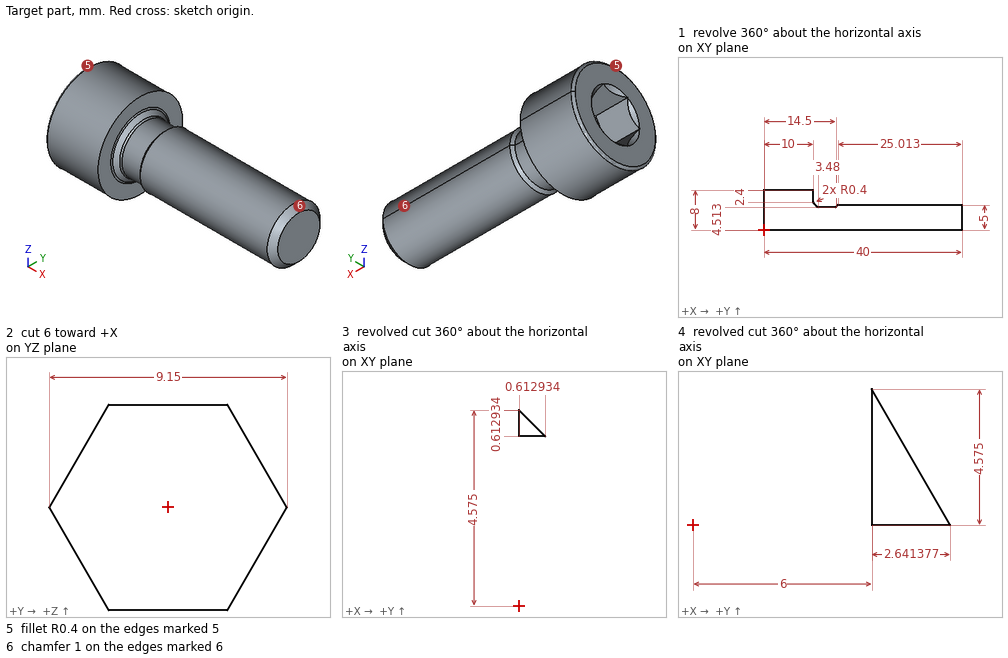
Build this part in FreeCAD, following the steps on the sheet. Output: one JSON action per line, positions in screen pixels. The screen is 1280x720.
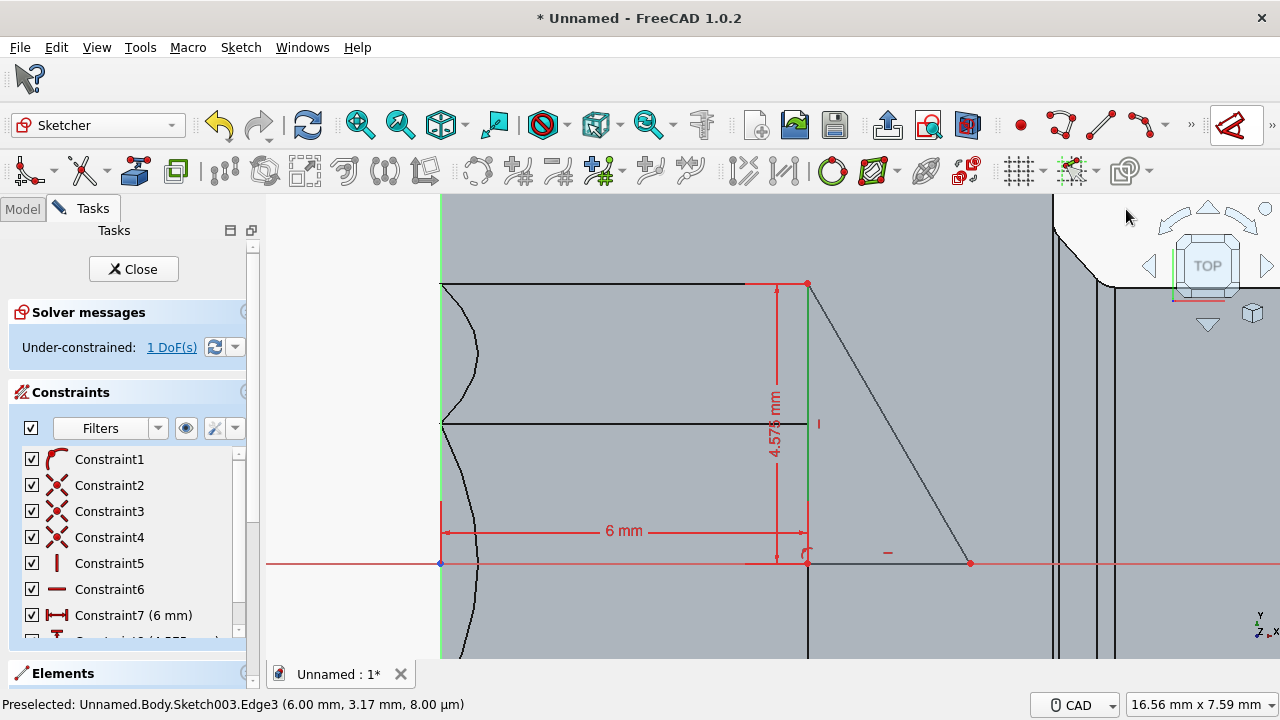
{"action": "left_click", "coordinate": [857, 564]}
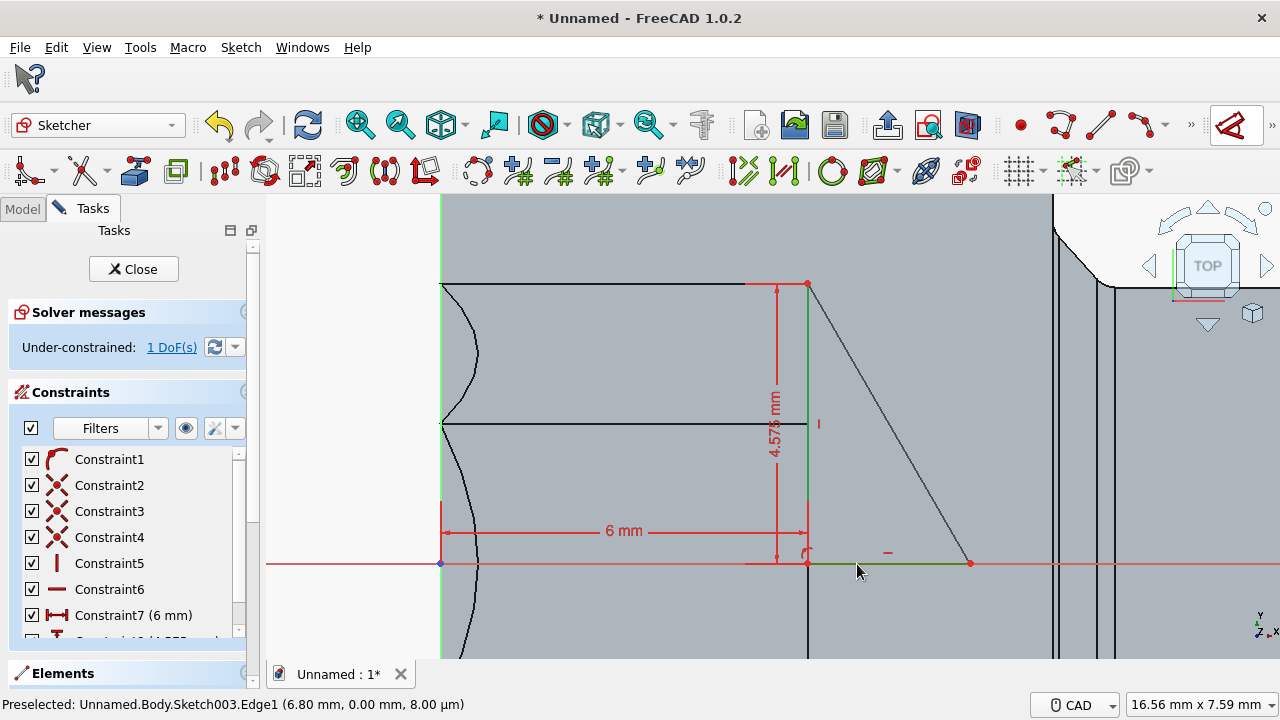
{"action": "left_click", "coordinate": [1258, 126]}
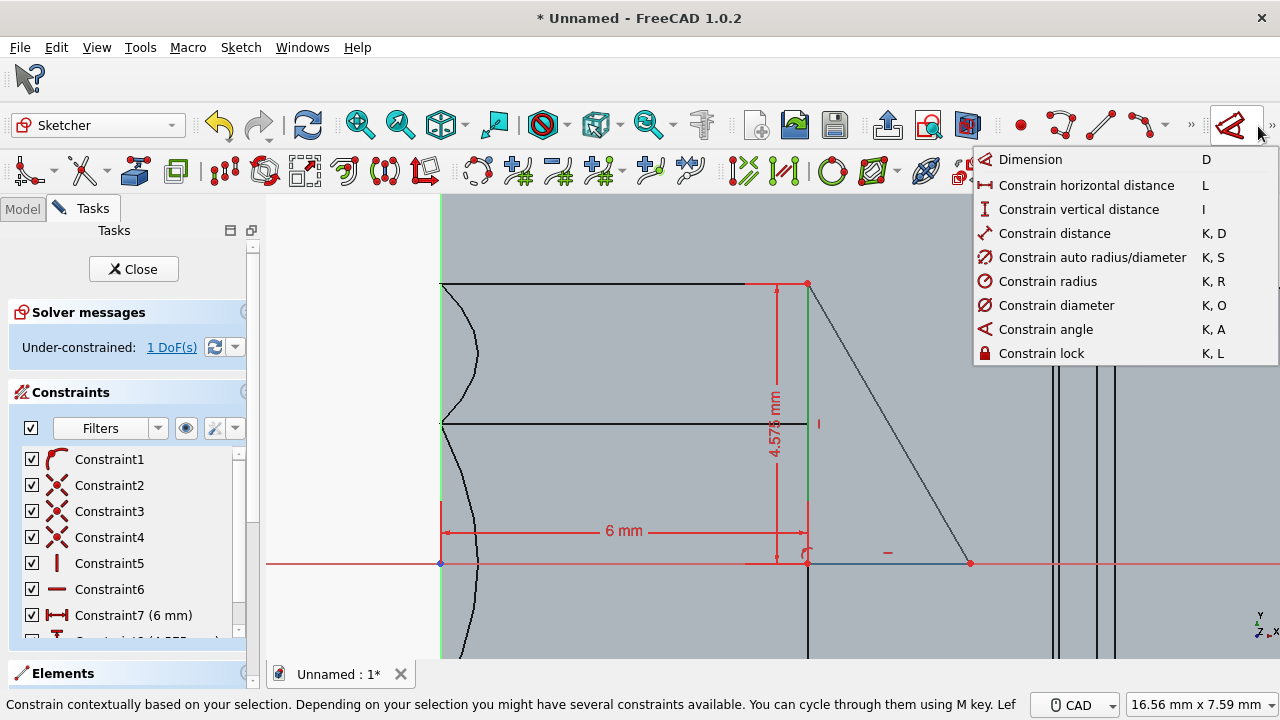
{"action": "left_click", "coordinate": [1126, 185]}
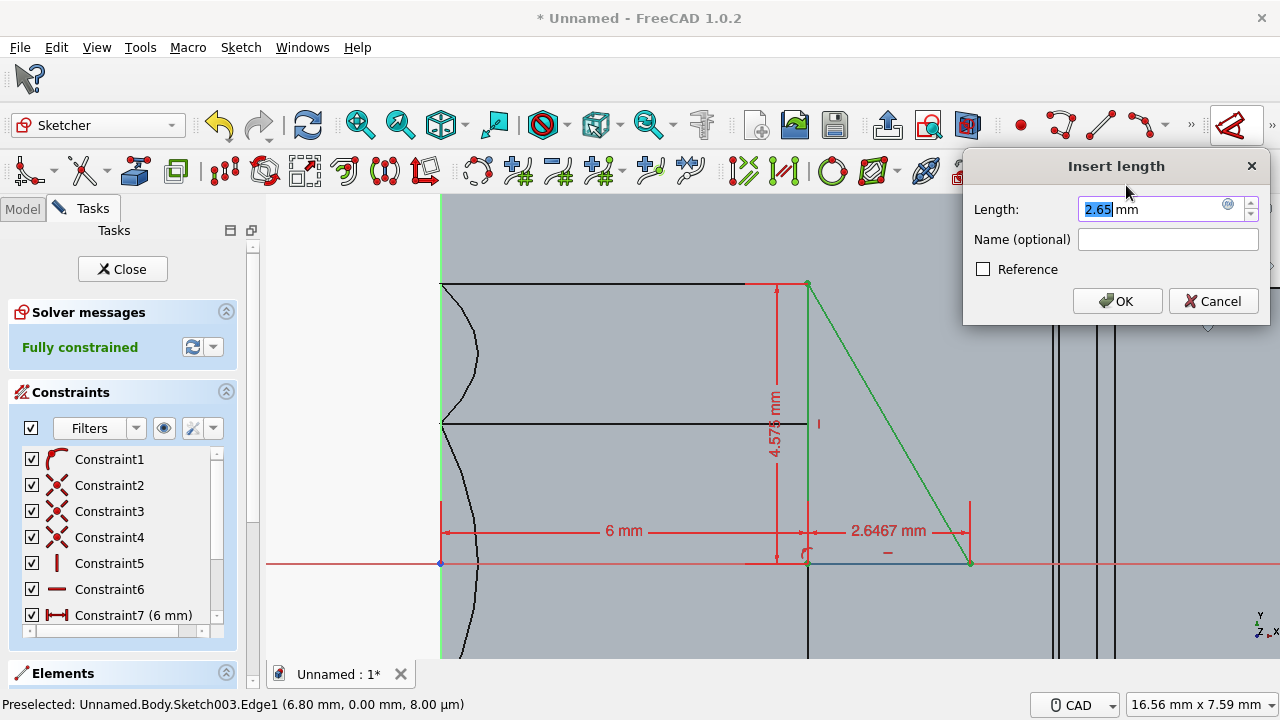
{"action": "type", "text": "2.641377"}
{"action": "key", "text": "Return"}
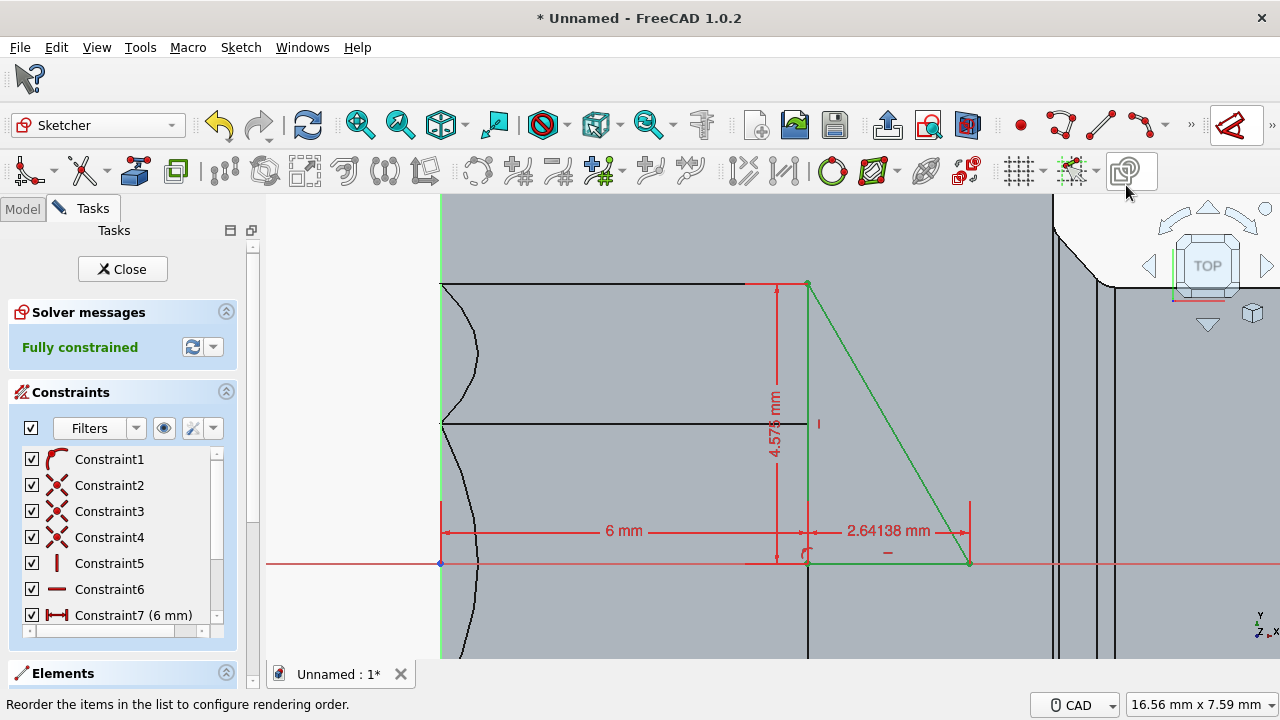
{"action": "left_click", "coordinate": [123, 269]}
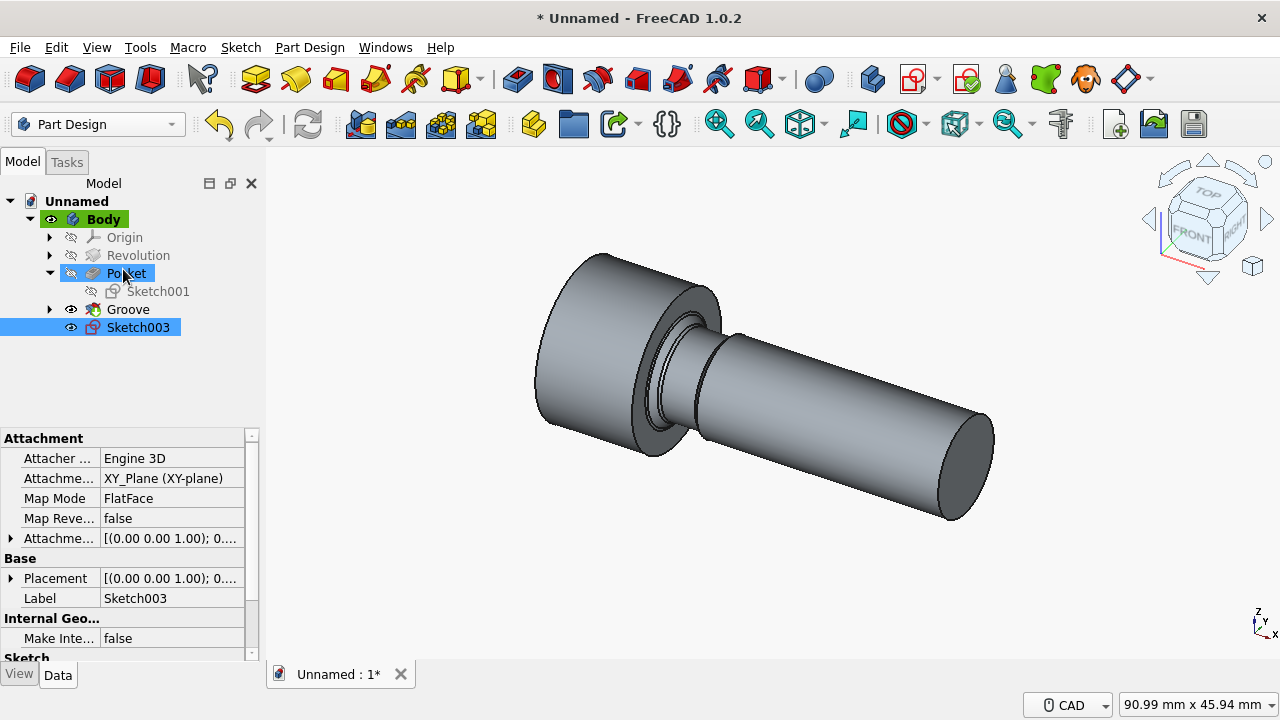
{"action": "left_click", "coordinate": [598, 80]}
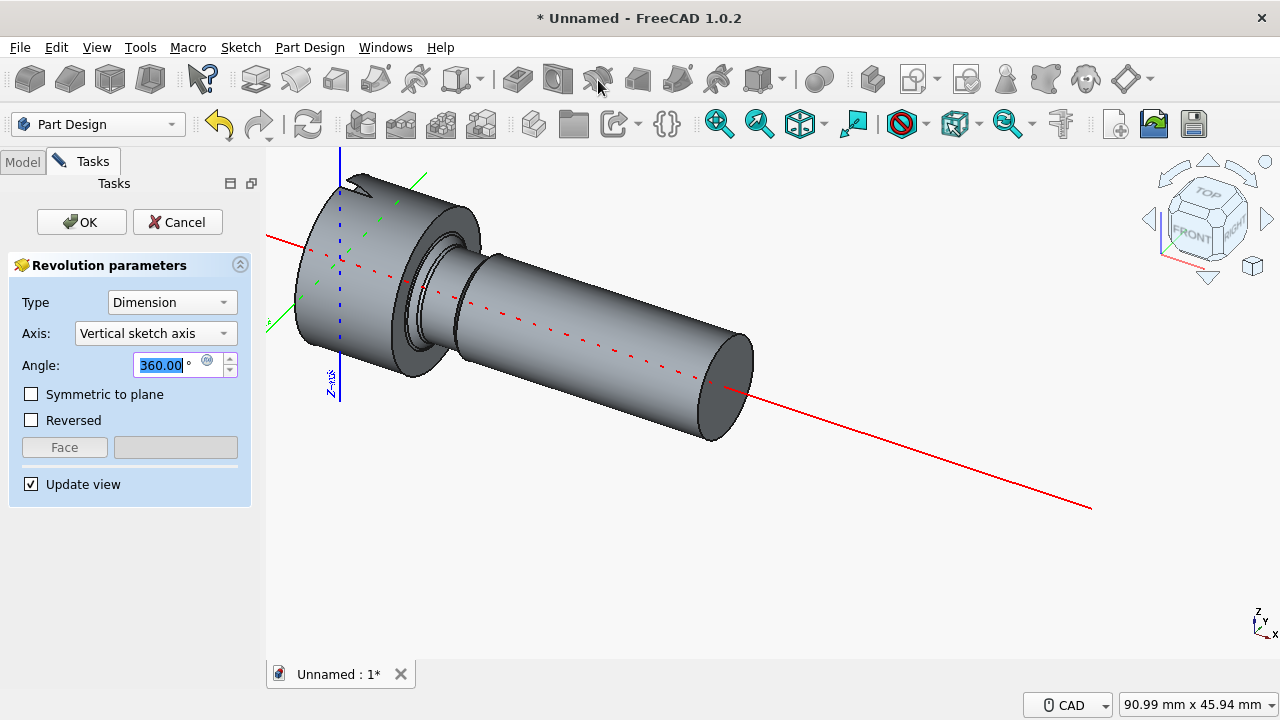
{"action": "left_click", "coordinate": [156, 334]}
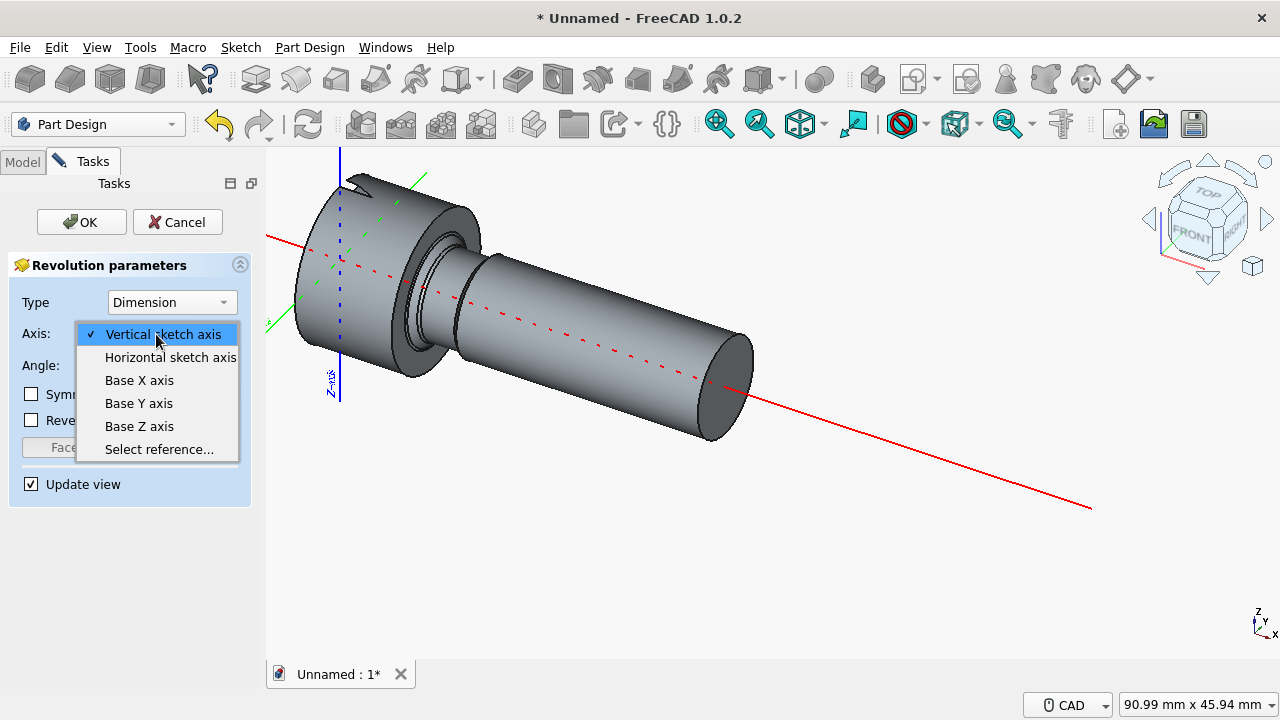
{"action": "left_click", "coordinate": [156, 358]}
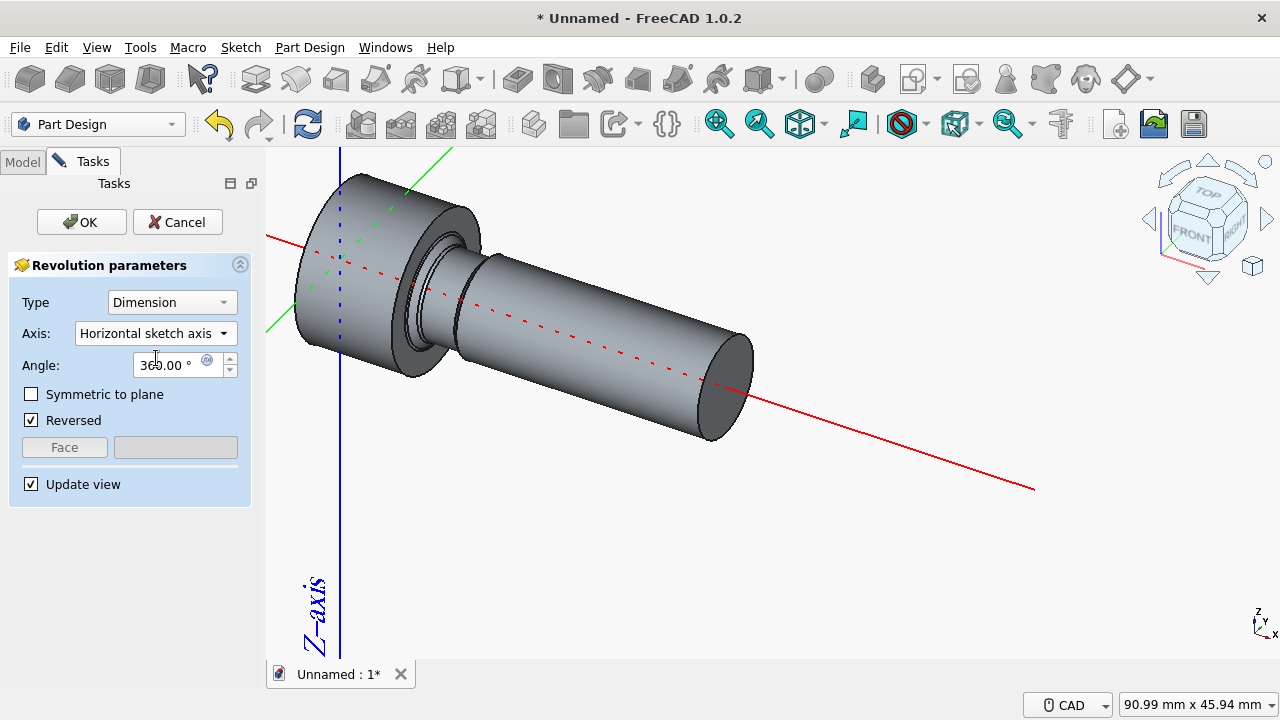
{"action": "left_click", "coordinate": [82, 222]}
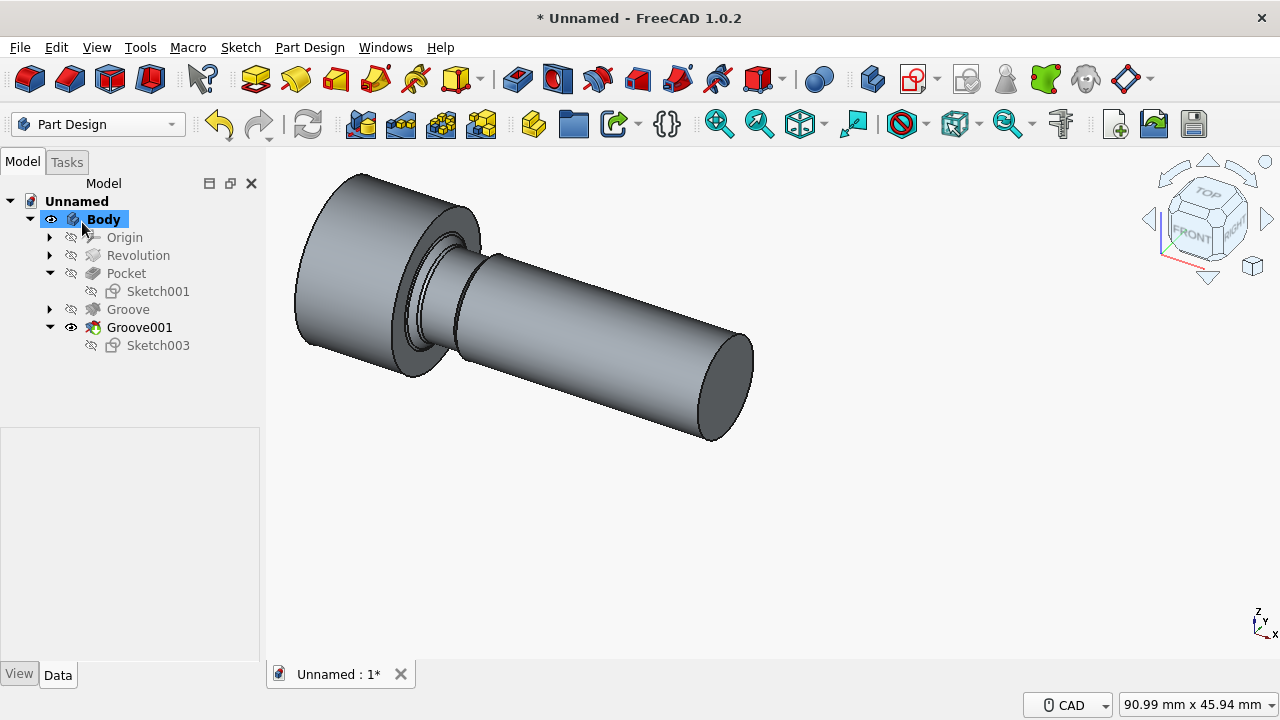
{"action": "left_click", "coordinate": [720, 124]}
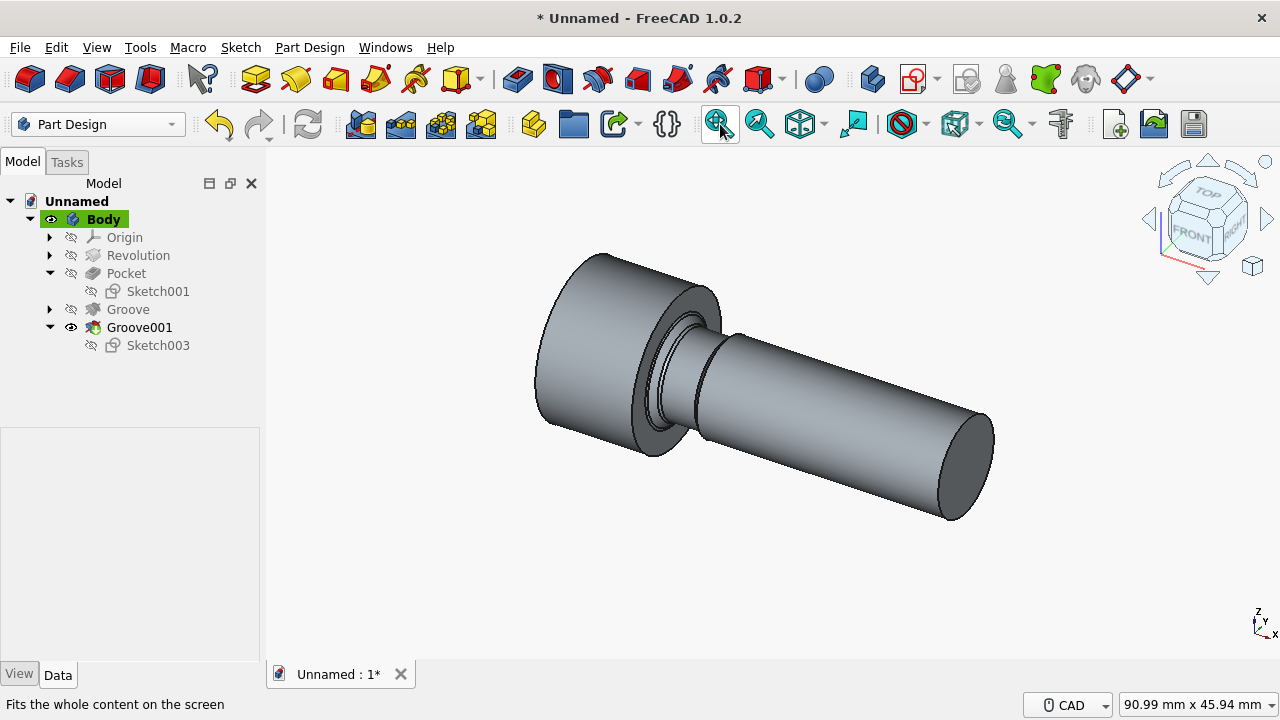
{"action": "key", "text": "0"}